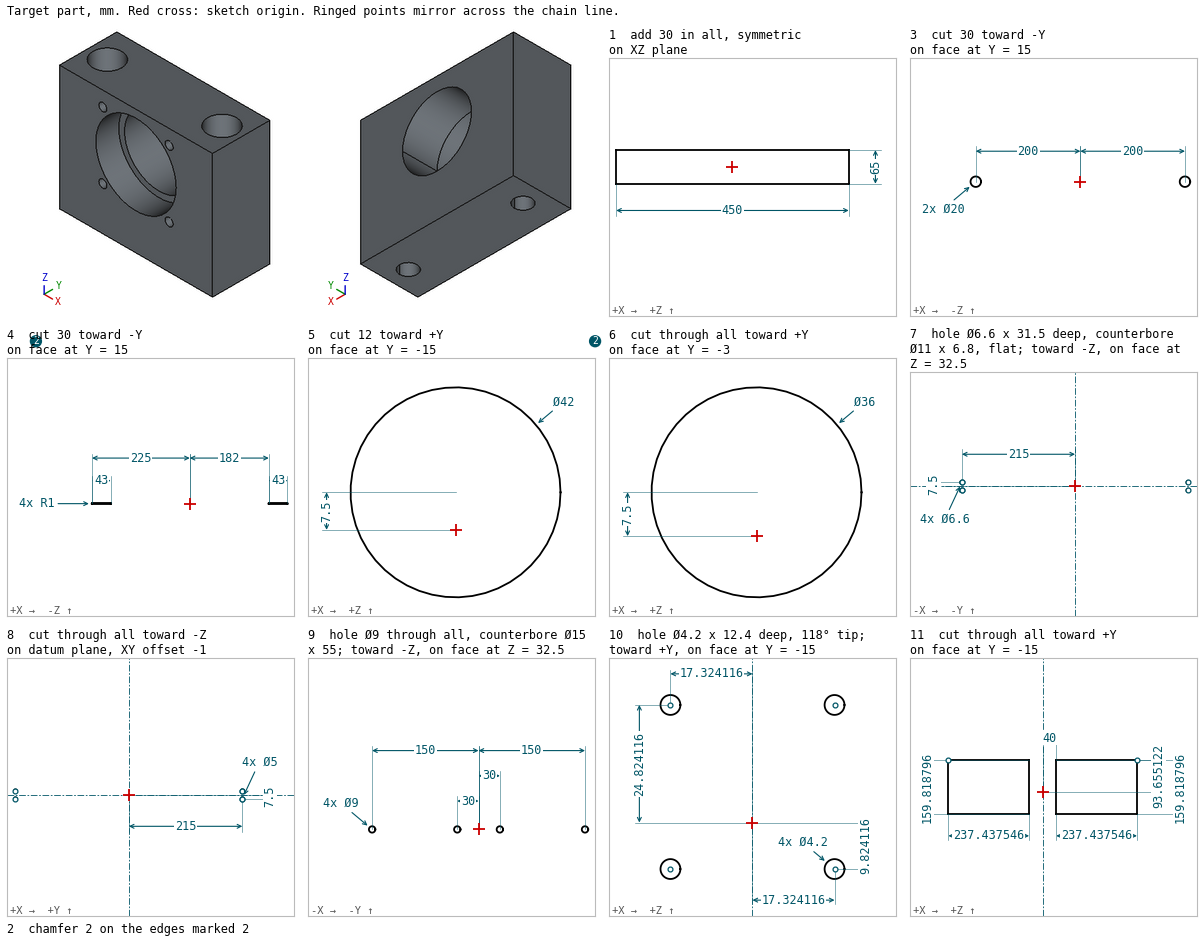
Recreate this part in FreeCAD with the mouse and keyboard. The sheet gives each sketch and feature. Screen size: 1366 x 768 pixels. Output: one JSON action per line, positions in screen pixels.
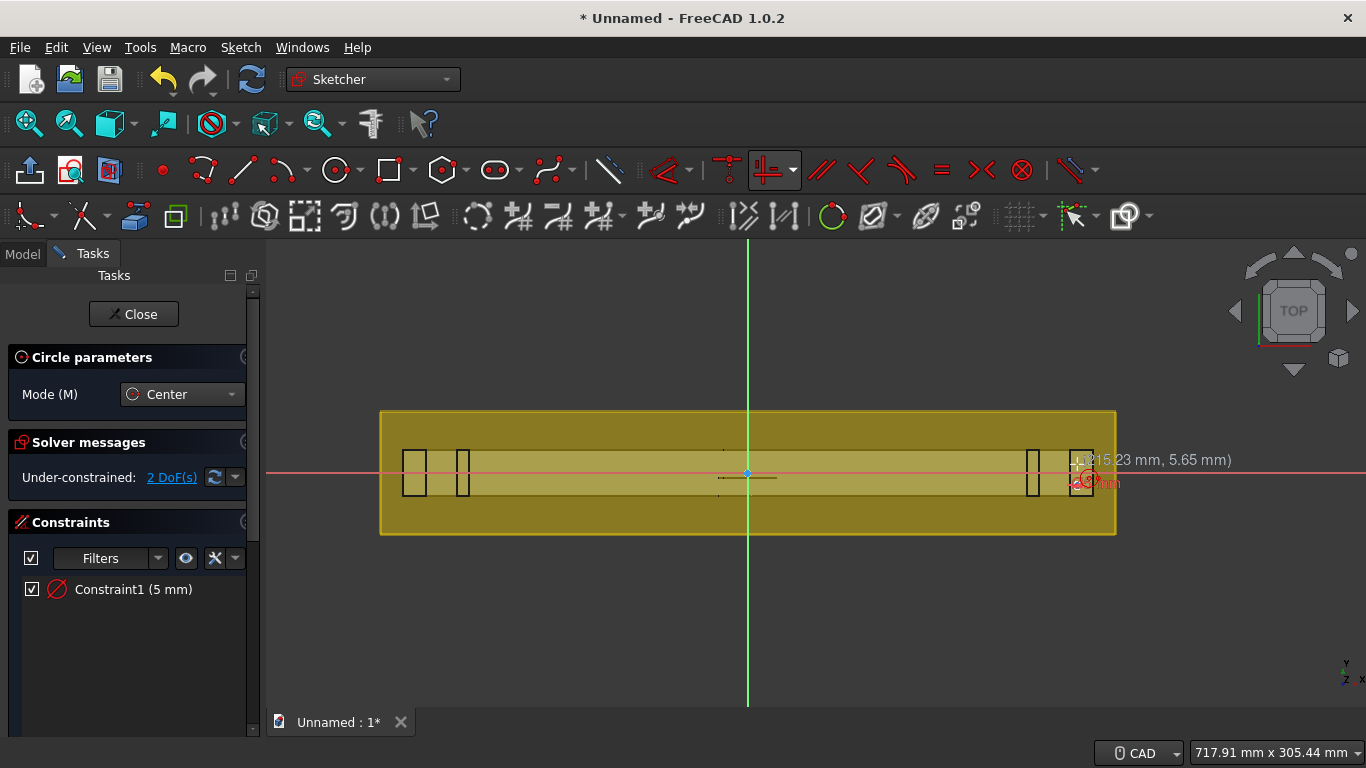
{"action": "scroll", "coordinate": [1077, 462], "scroll_direction": "up", "scroll_amount": 2}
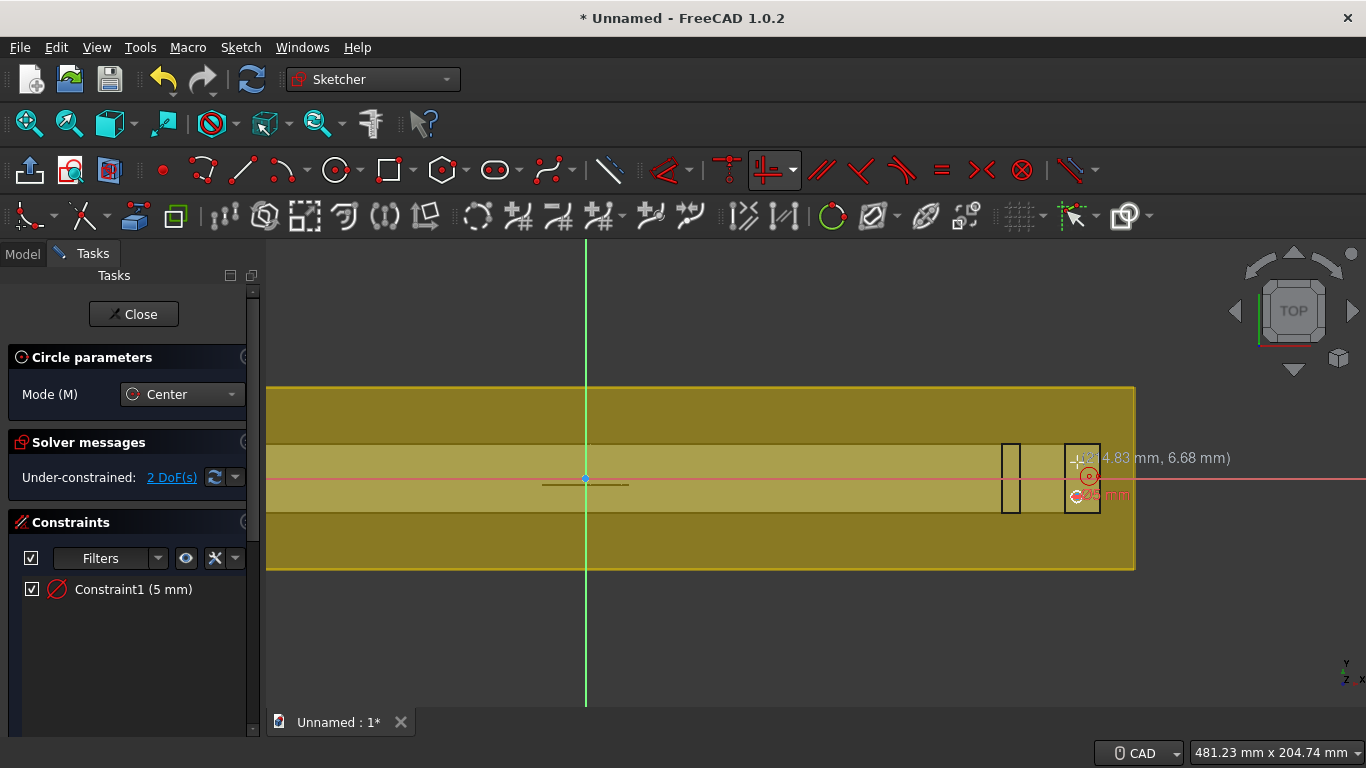
{"action": "left_click", "coordinate": [1077, 461]}
{"action": "mouse_move", "coordinate": [1081, 457]}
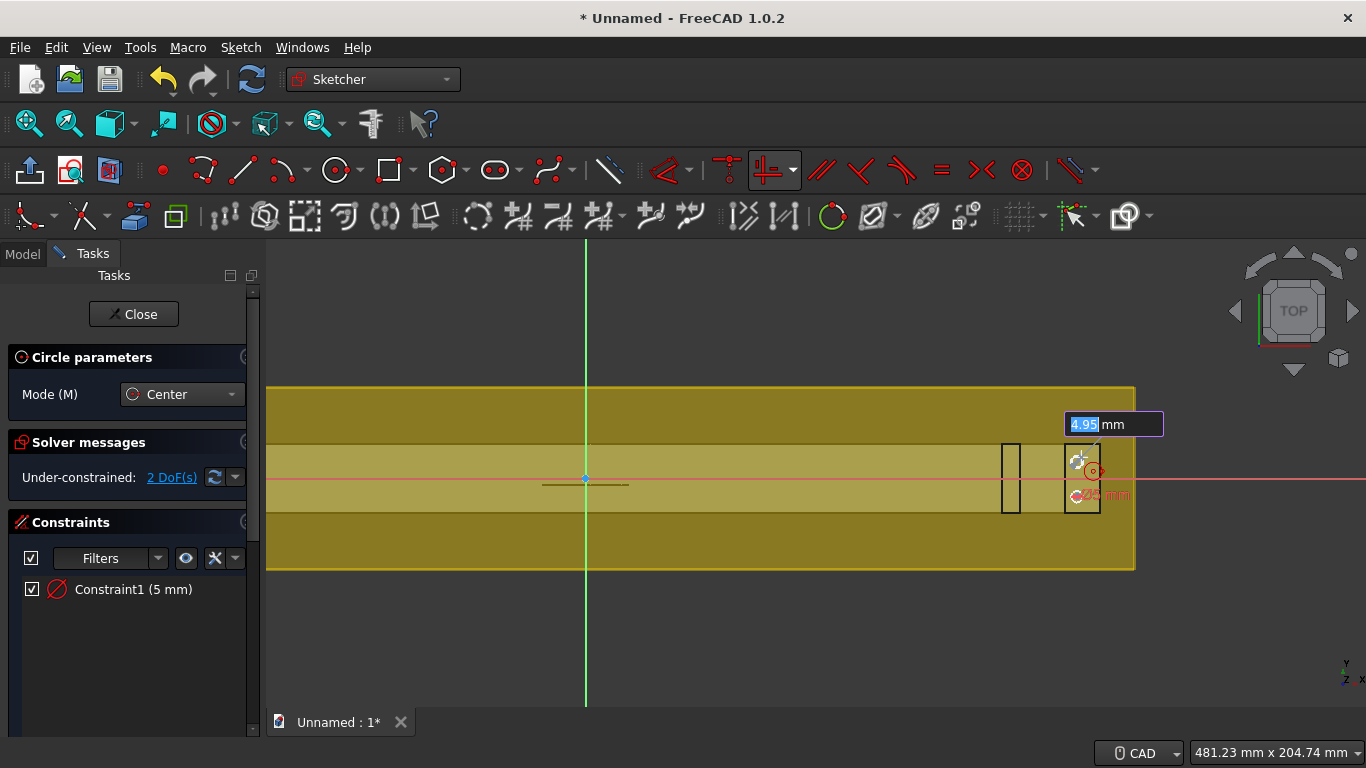
{"action": "type", "text": "5"}
{"action": "key", "text": "Return"}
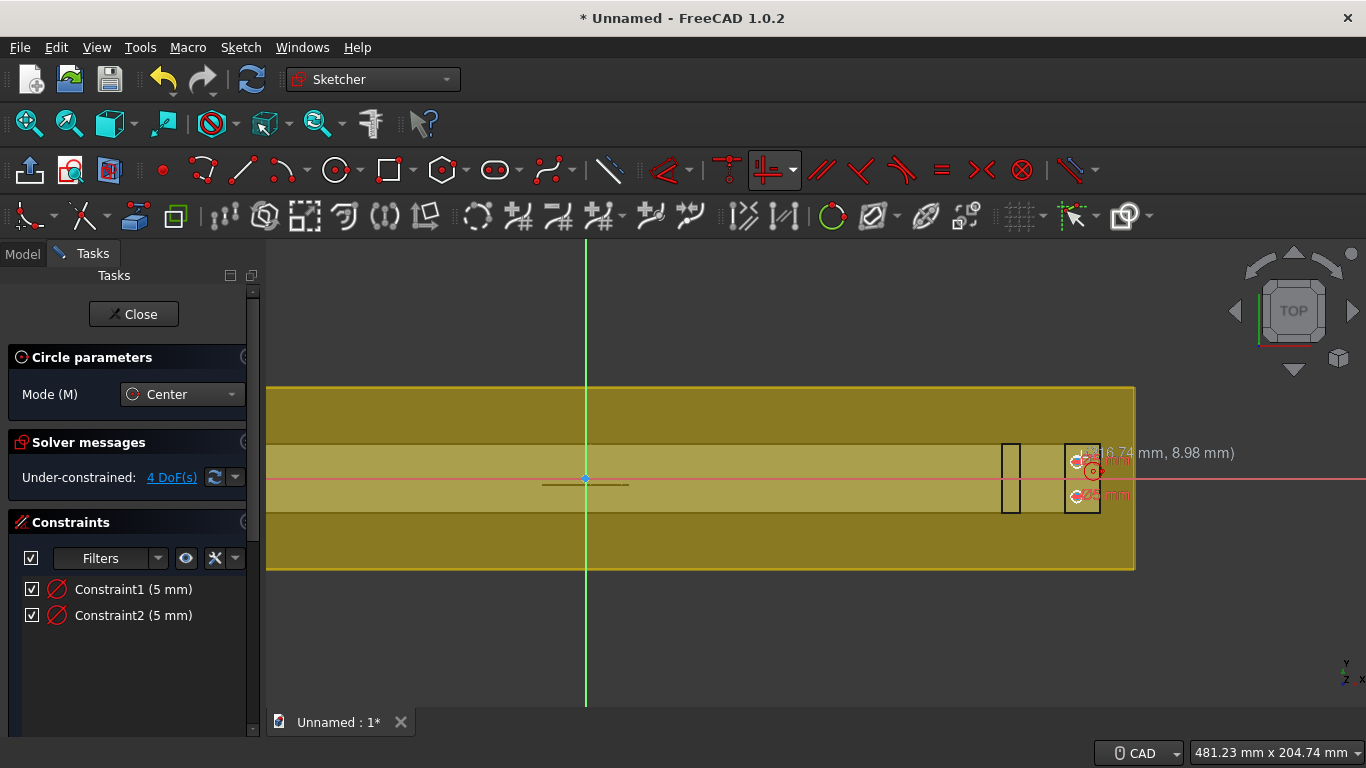
{"action": "scroll", "coordinate": [1077, 462], "scroll_direction": "down", "scroll_amount": 2}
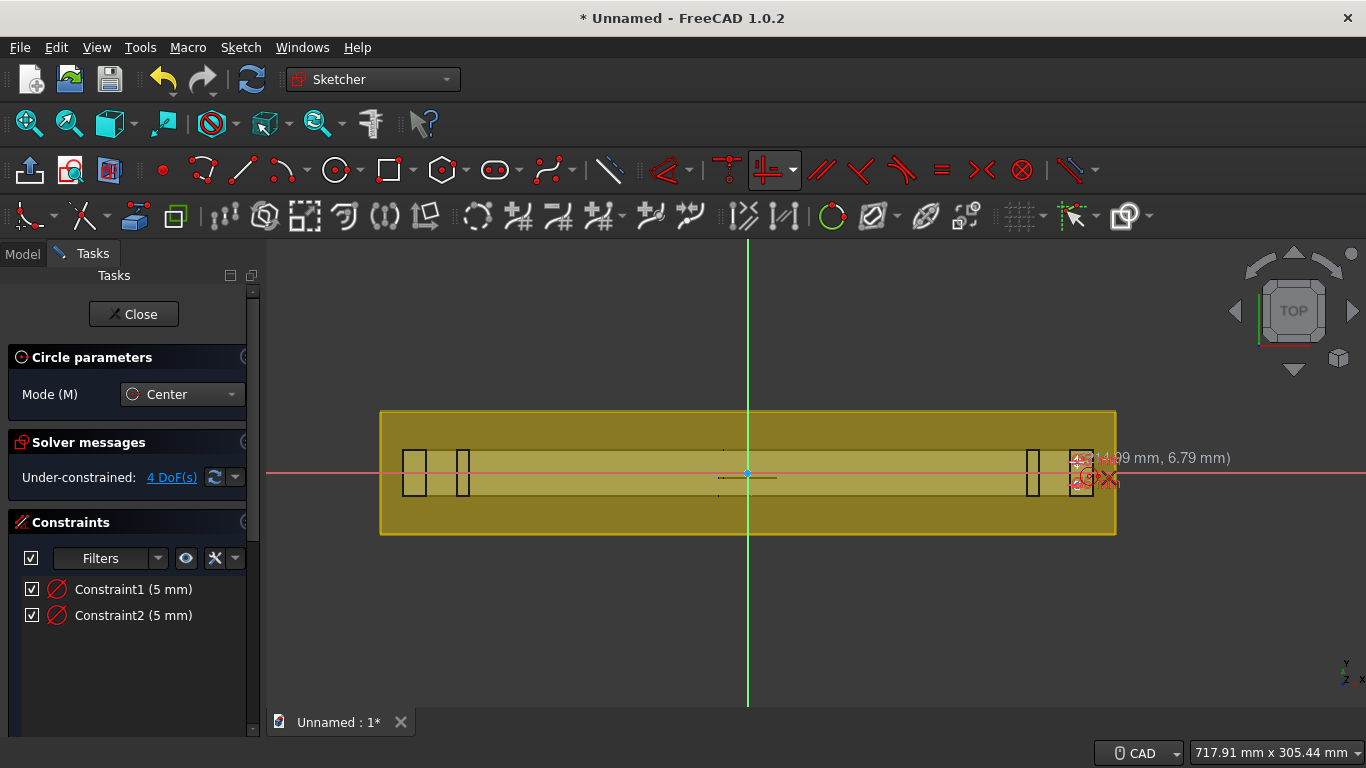
{"action": "scroll", "coordinate": [418, 485], "scroll_direction": "up", "scroll_amount": 9}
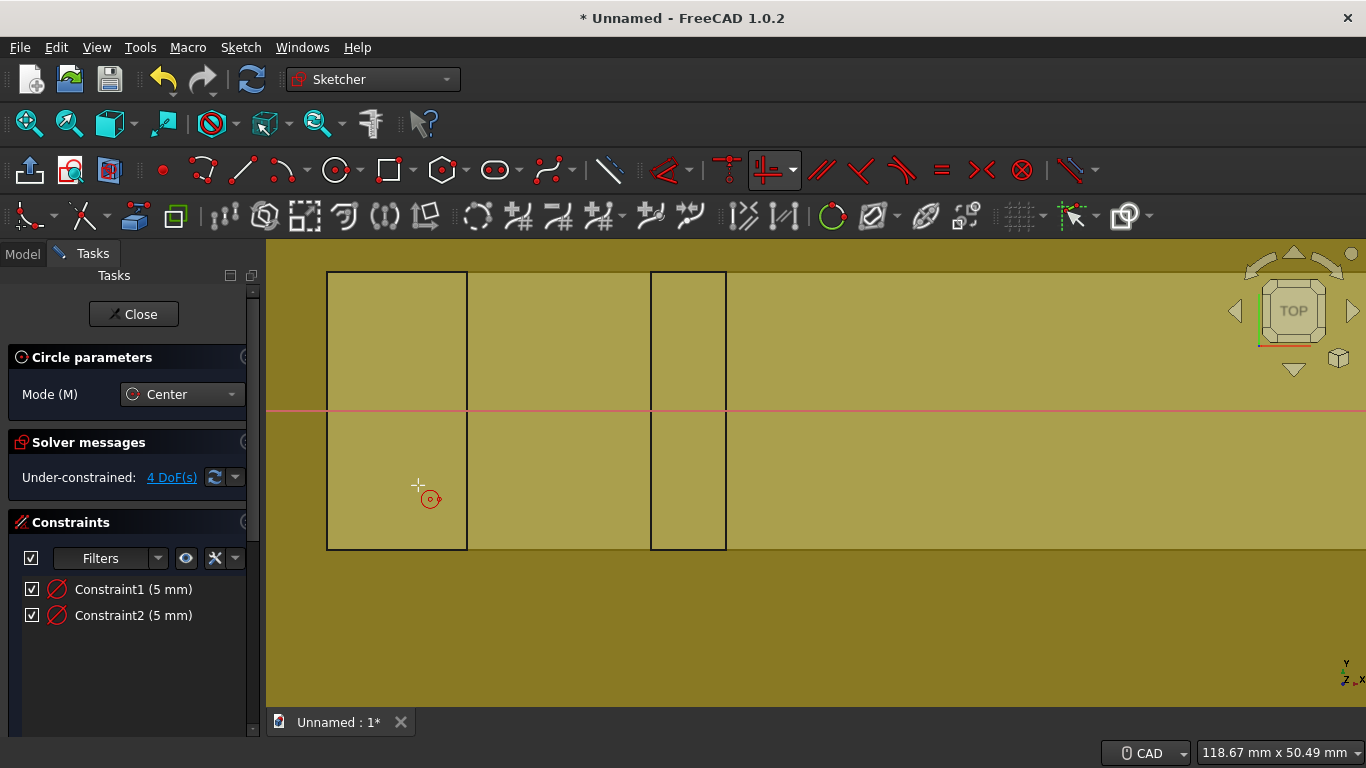
{"action": "scroll", "coordinate": [418, 485], "scroll_direction": "down", "scroll_amount": 9}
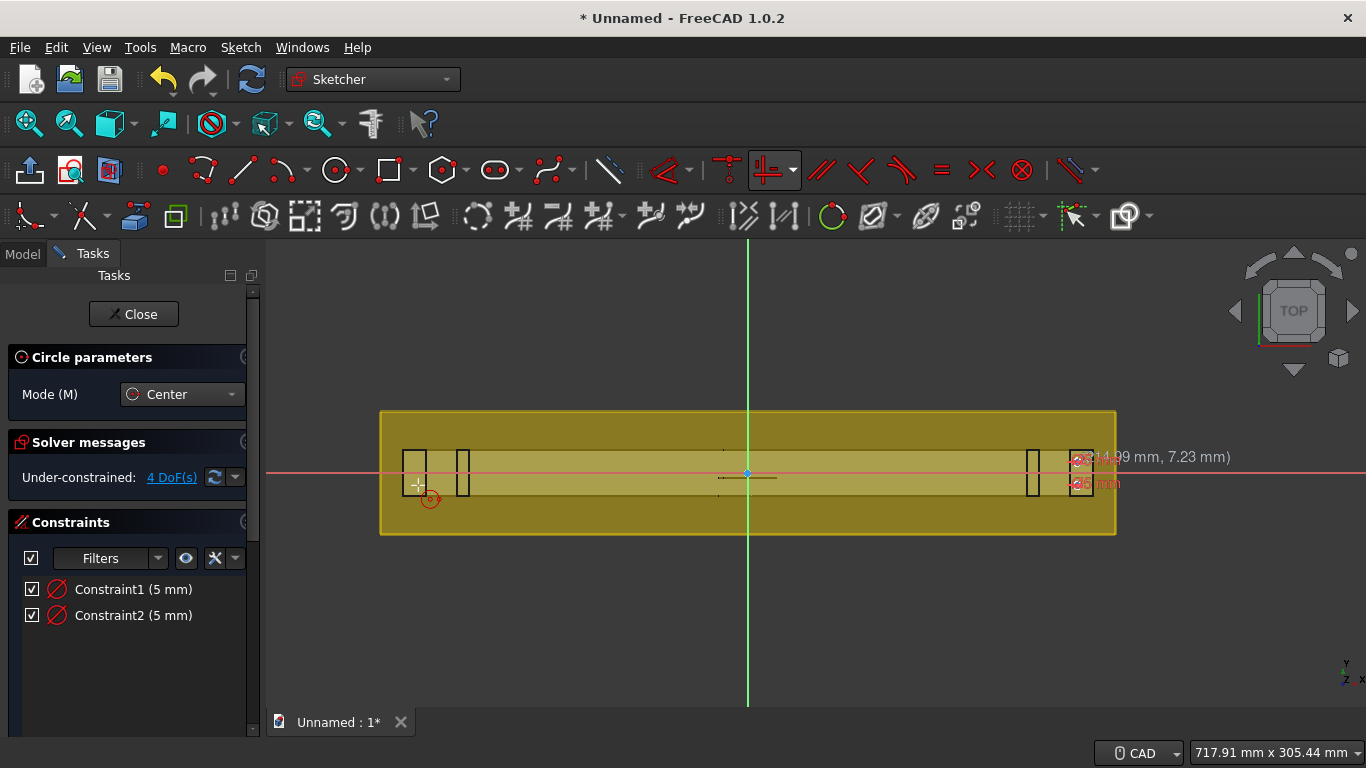
{"action": "scroll", "coordinate": [418, 485], "scroll_direction": "up", "scroll_amount": 2}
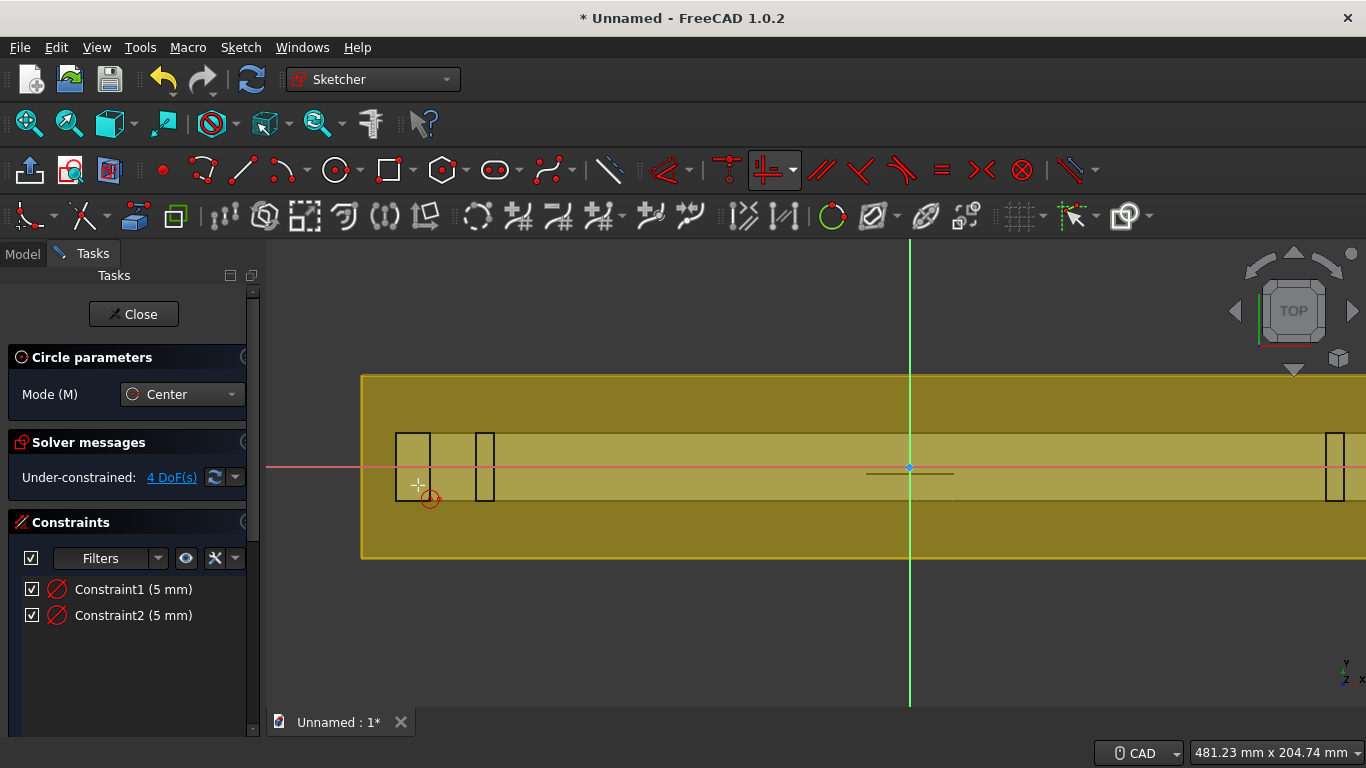
{"action": "left_click", "coordinate": [419, 484]}
{"action": "mouse_move", "coordinate": [423, 488]}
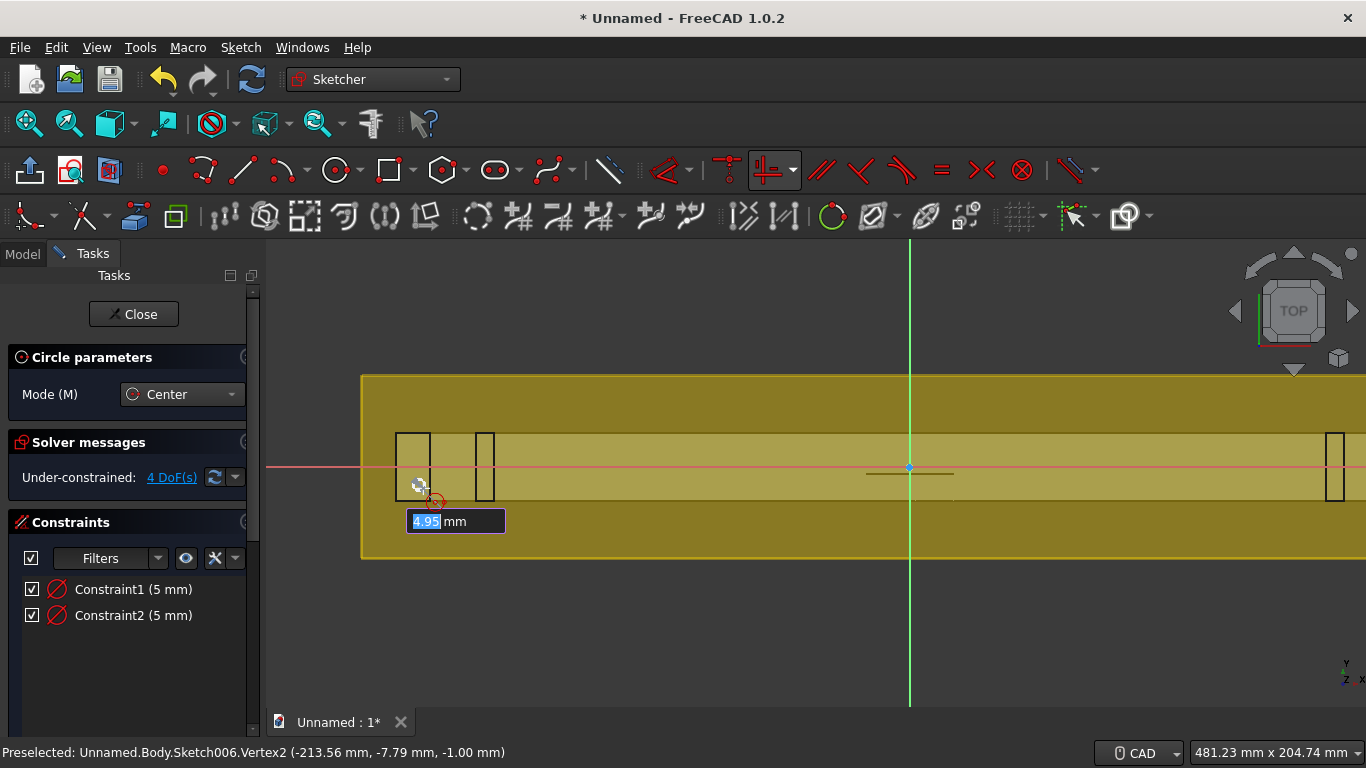
{"action": "type", "text": "5"}
{"action": "key", "text": "Return"}